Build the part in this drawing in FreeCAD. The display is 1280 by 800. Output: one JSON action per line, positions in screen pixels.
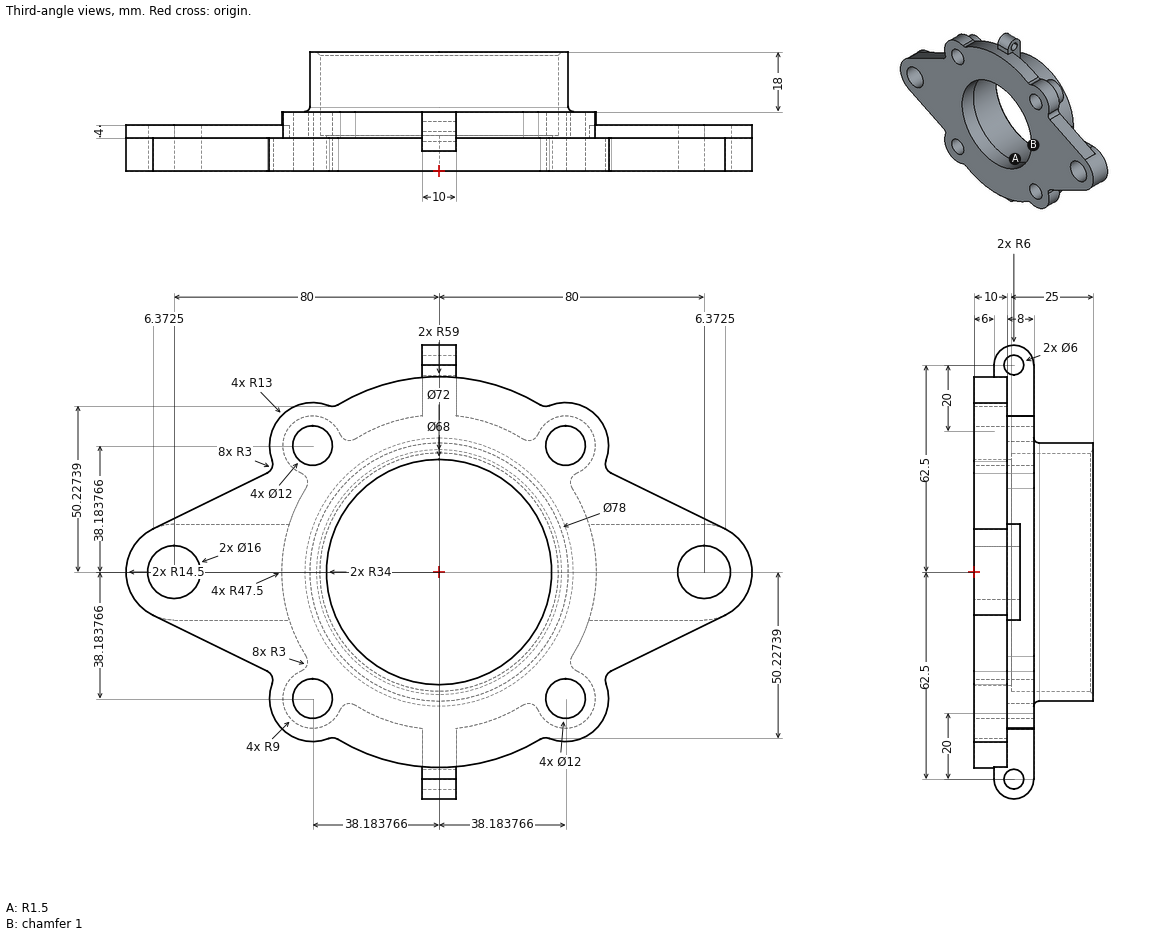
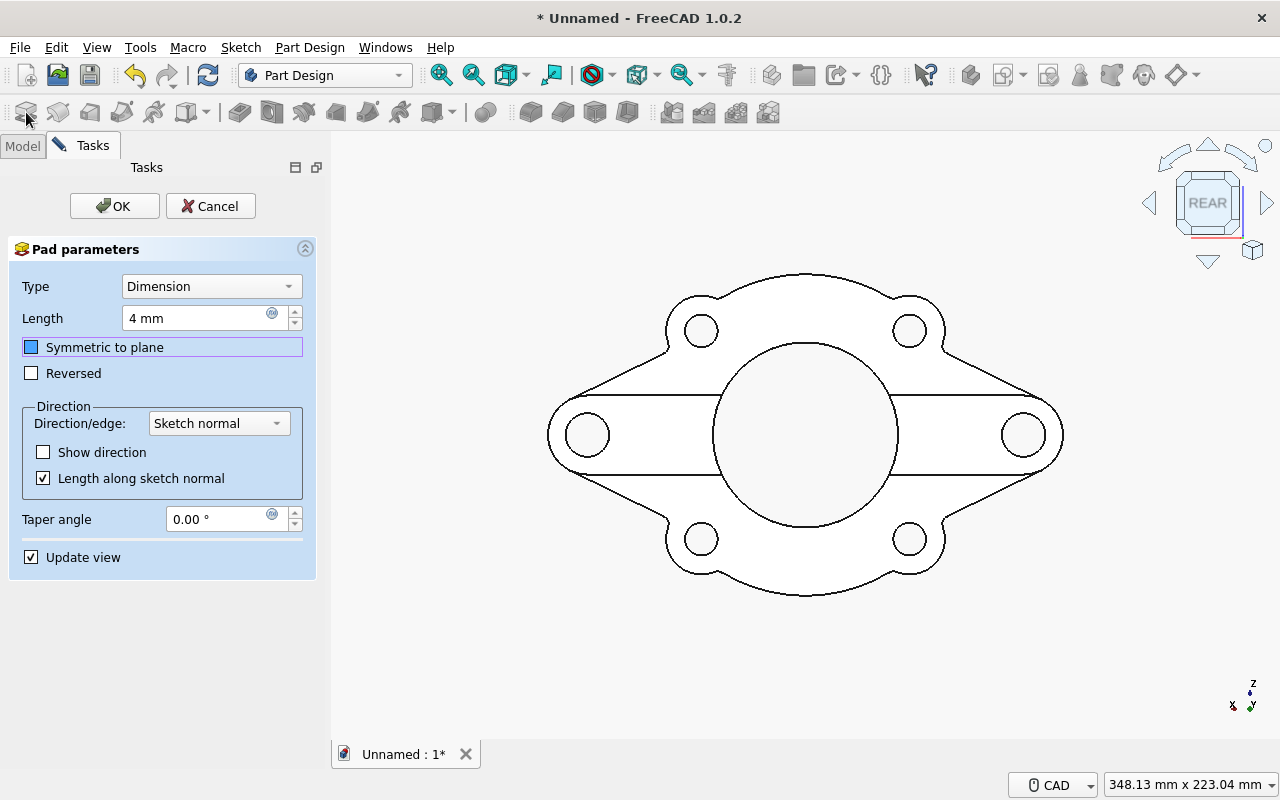
{"action": "left_click", "coordinate": [115, 206]}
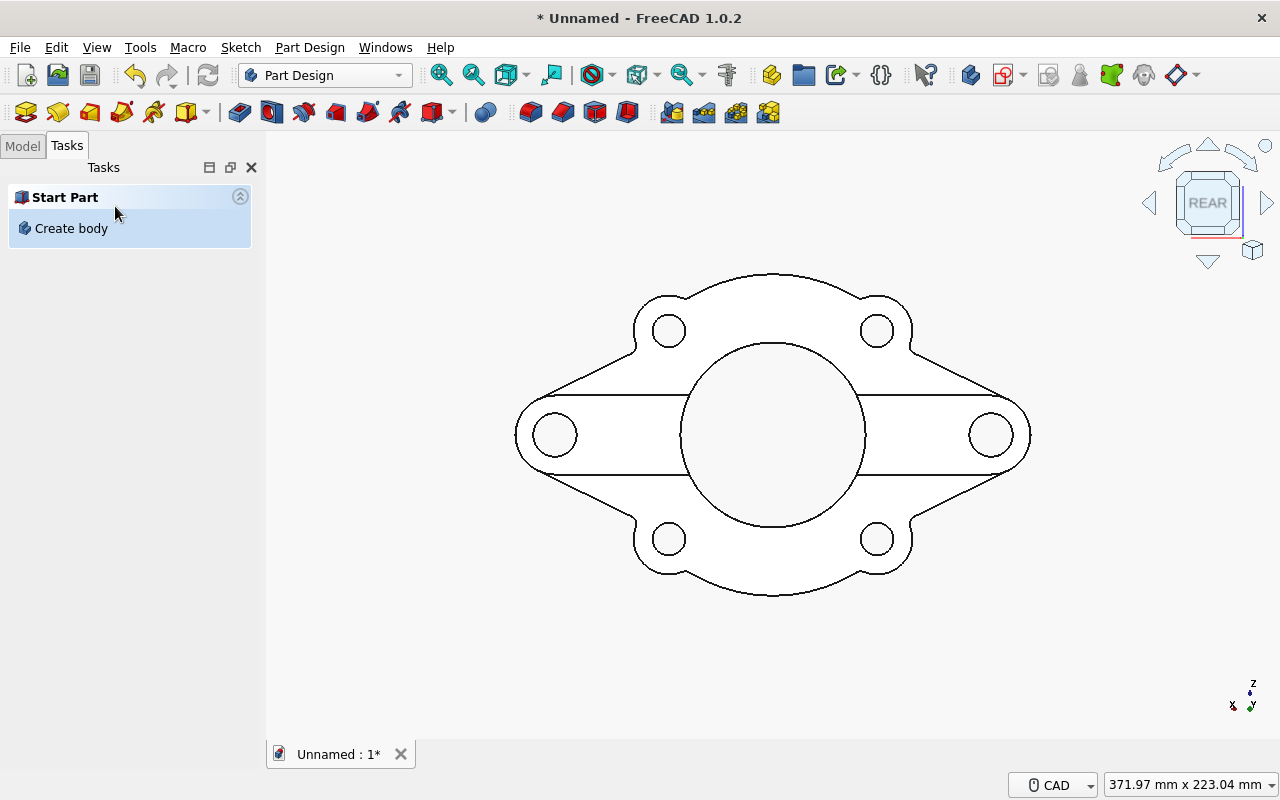
{"action": "left_click", "coordinate": [773, 300]}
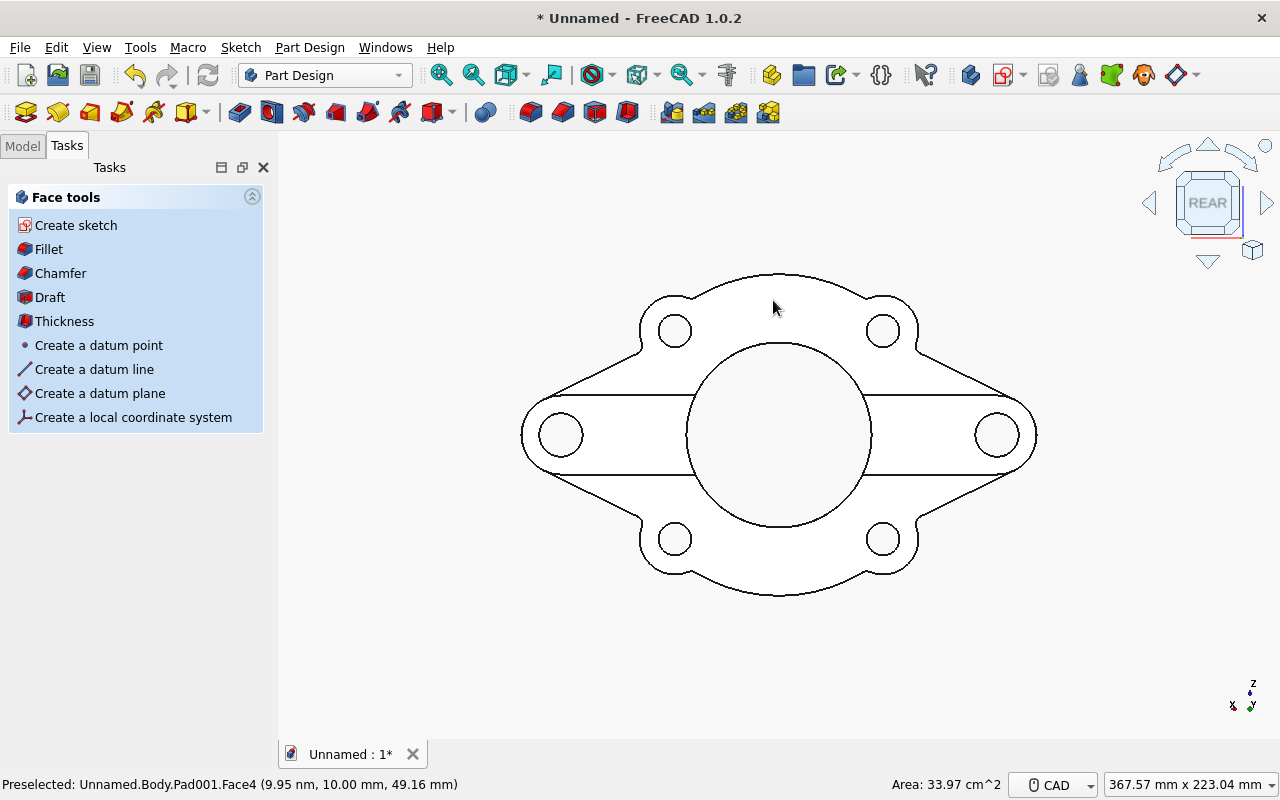
{"action": "left_click", "coordinate": [1004, 76]}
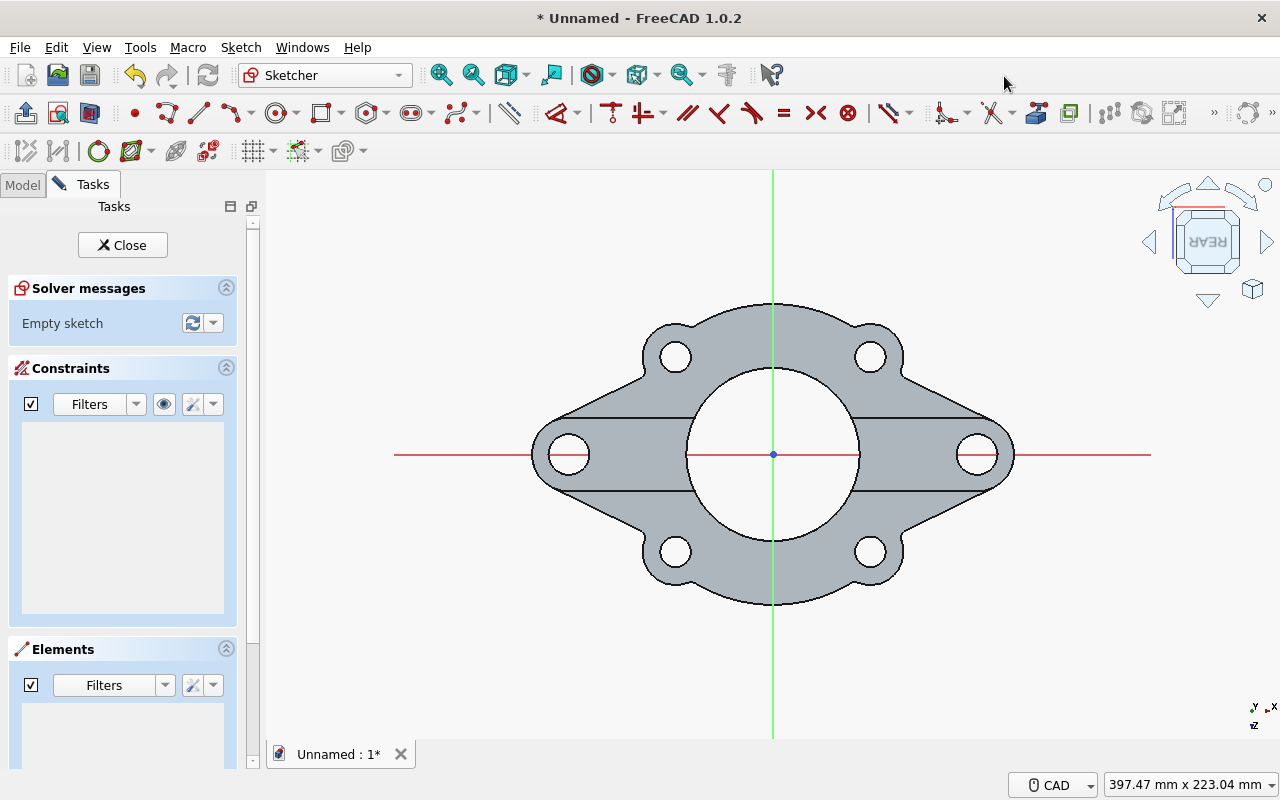
{"action": "left_click", "coordinate": [90, 114]}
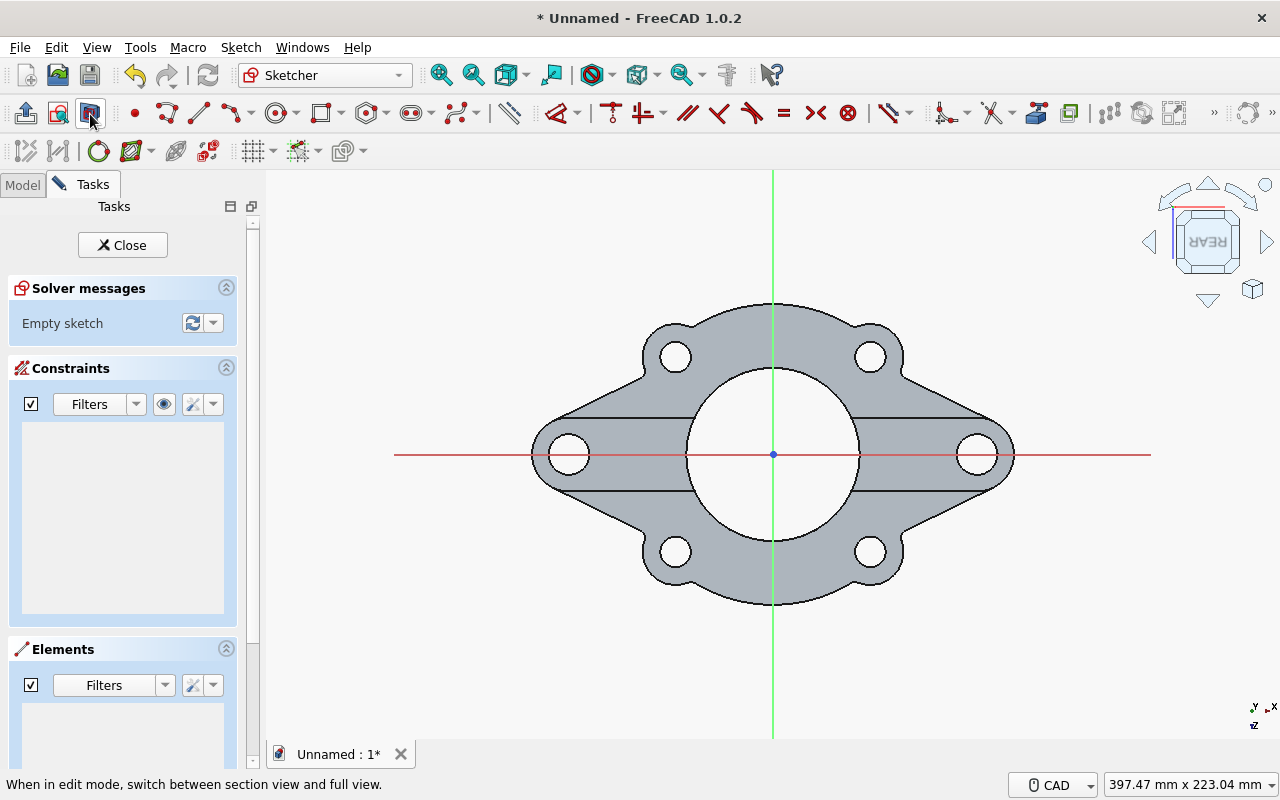
{"action": "scroll", "coordinate": [912, 454], "scroll_direction": "up", "scroll_amount": 2}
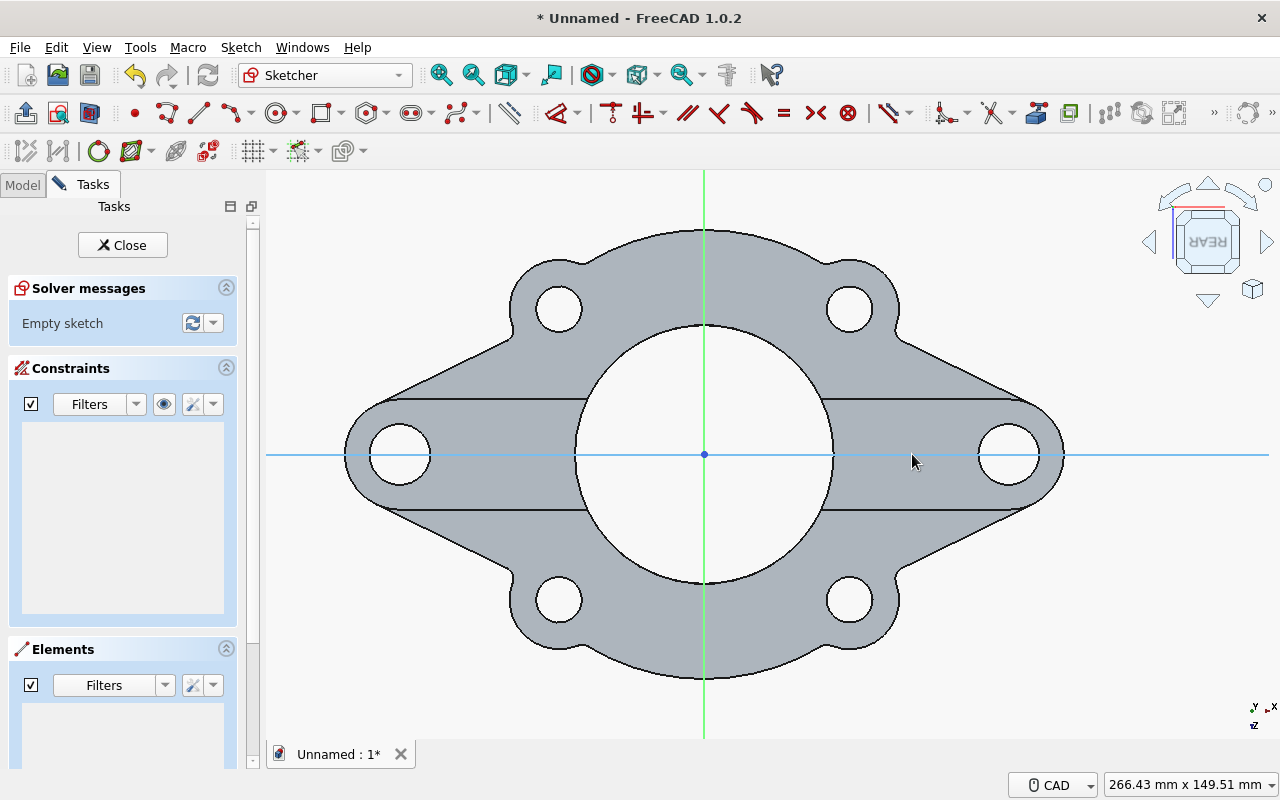
{"action": "left_click", "coordinate": [232, 114]}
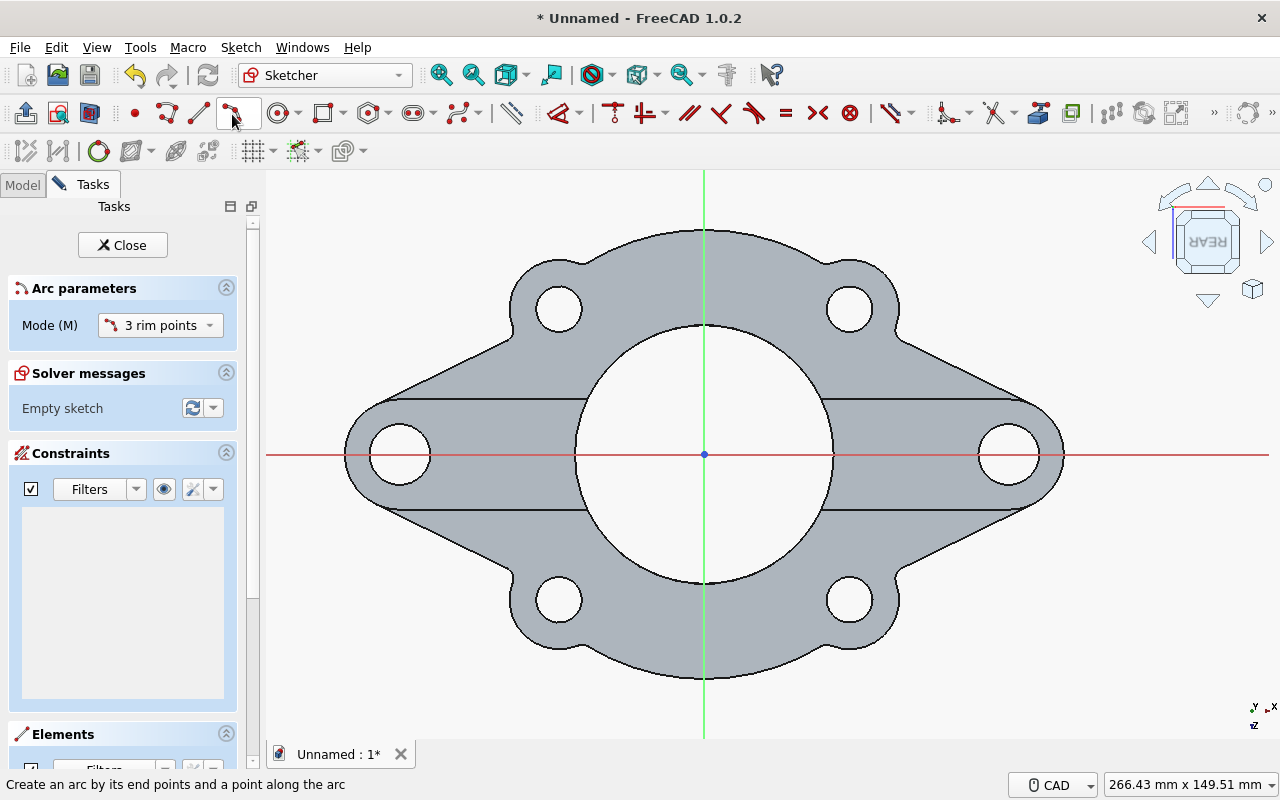
{"action": "left_click", "coordinate": [552, 358]}
{"action": "left_click", "coordinate": [552, 551]}
{"action": "left_click", "coordinate": [525, 434]}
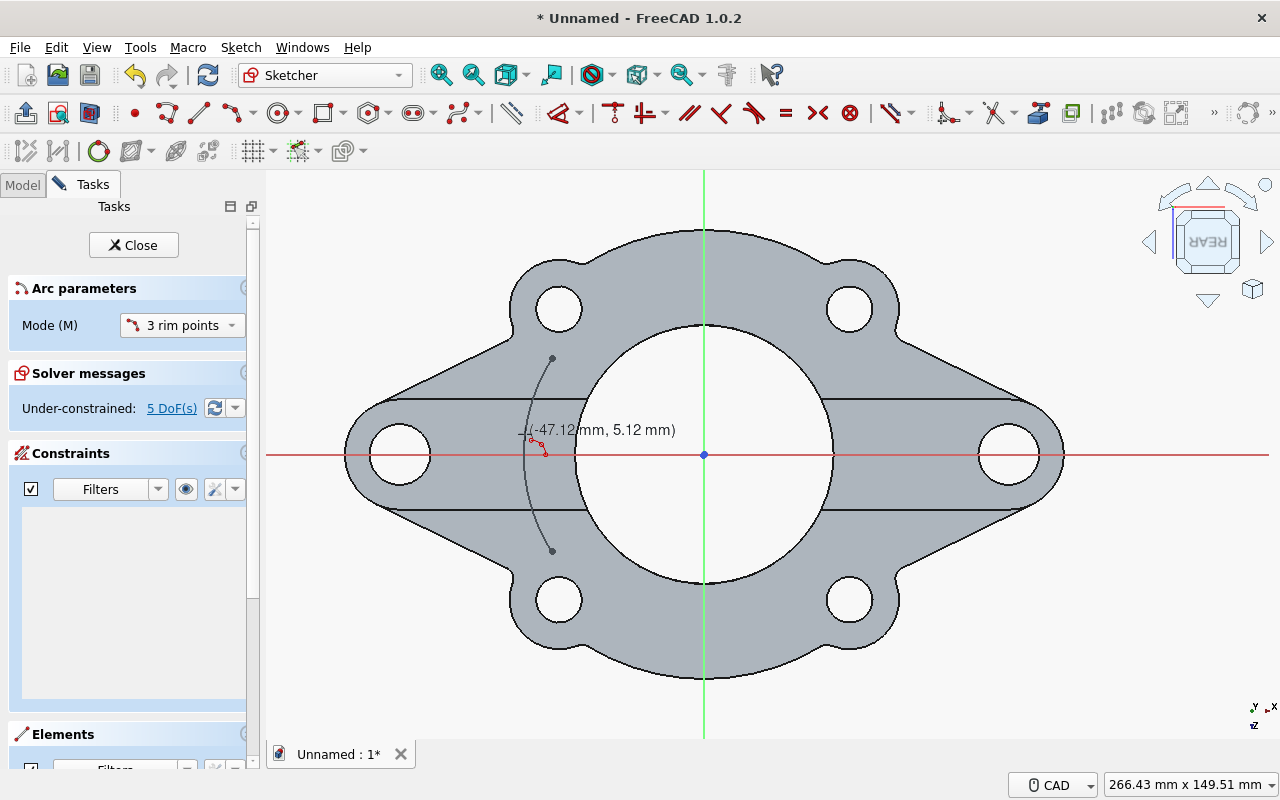
{"action": "left_click", "coordinate": [552, 552]}
{"action": "left_click", "coordinate": [546, 568]}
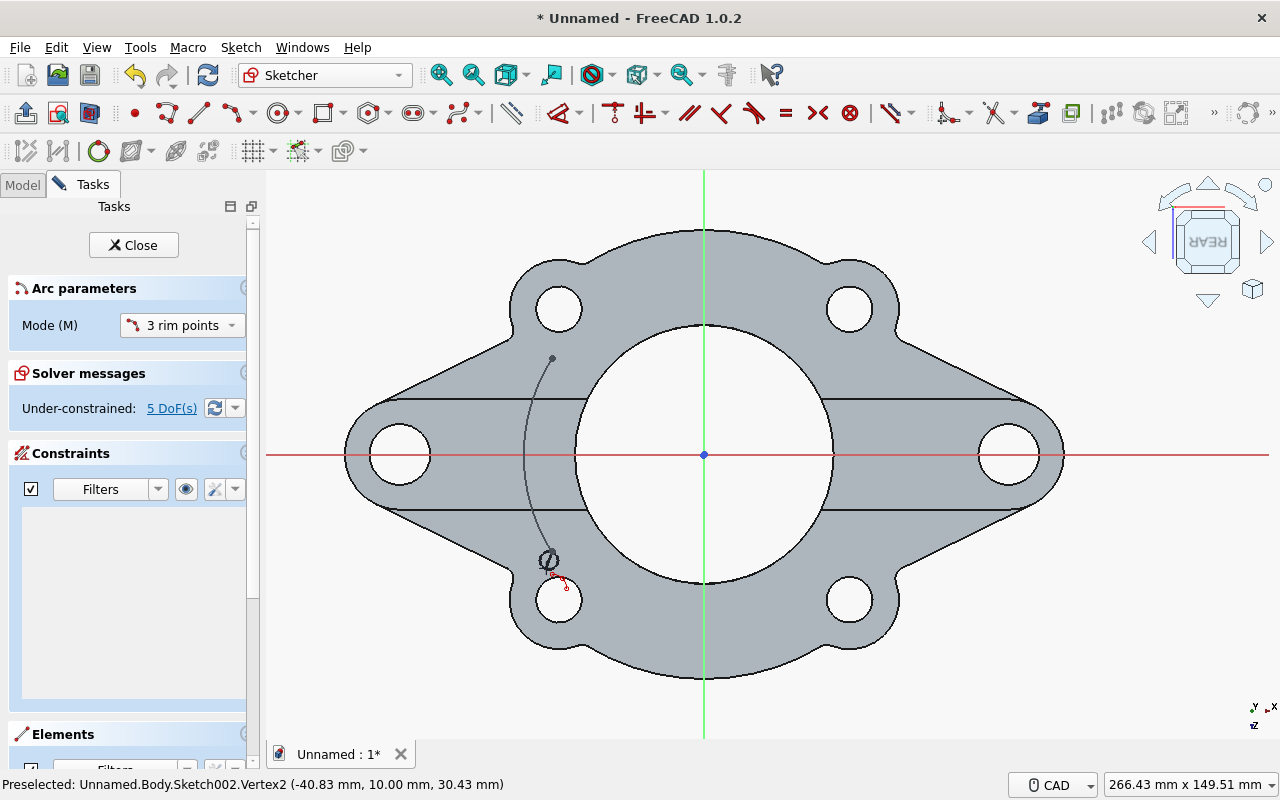
{"action": "scroll", "coordinate": [553, 561], "scroll_direction": "up", "scroll_amount": 7}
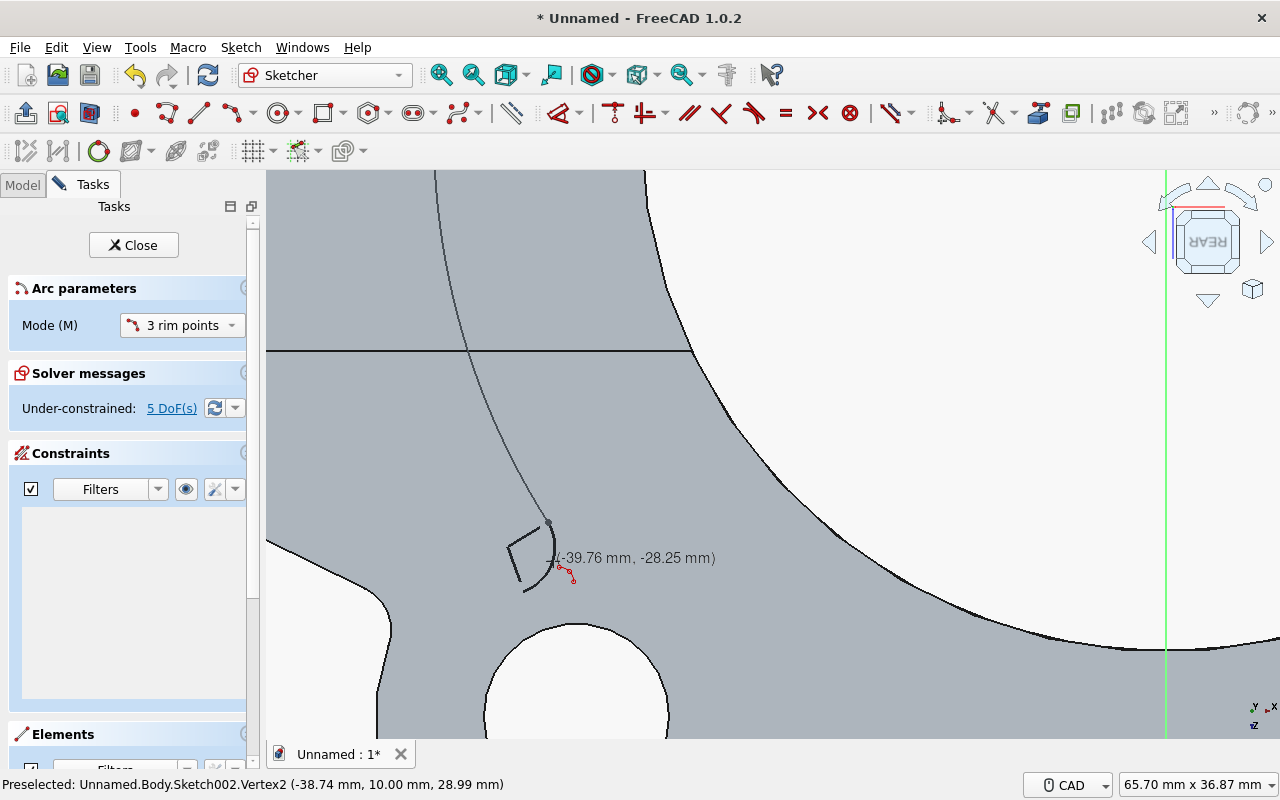
{"action": "left_click", "coordinate": [552, 559]}